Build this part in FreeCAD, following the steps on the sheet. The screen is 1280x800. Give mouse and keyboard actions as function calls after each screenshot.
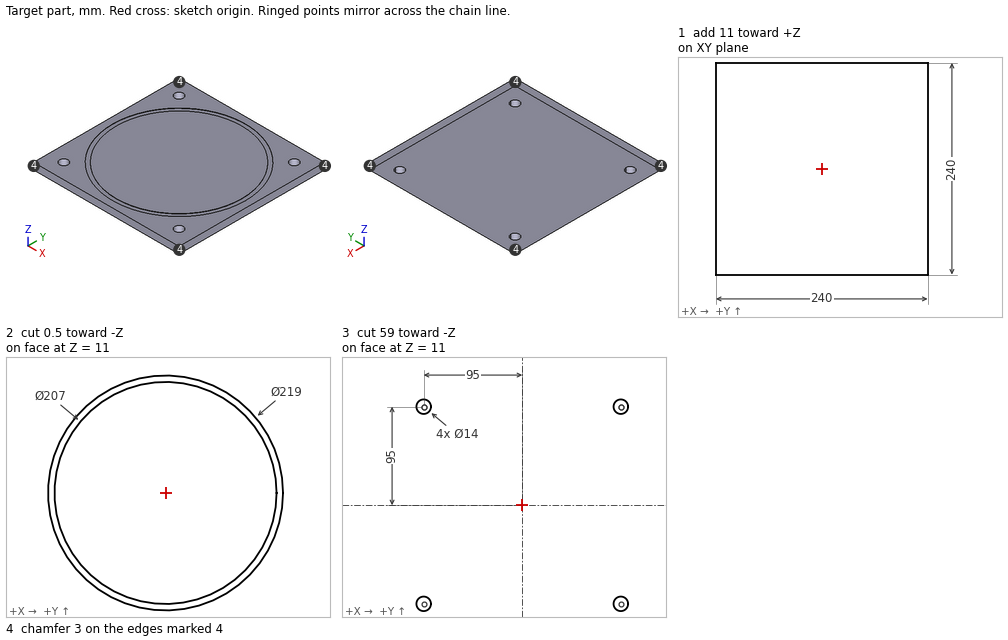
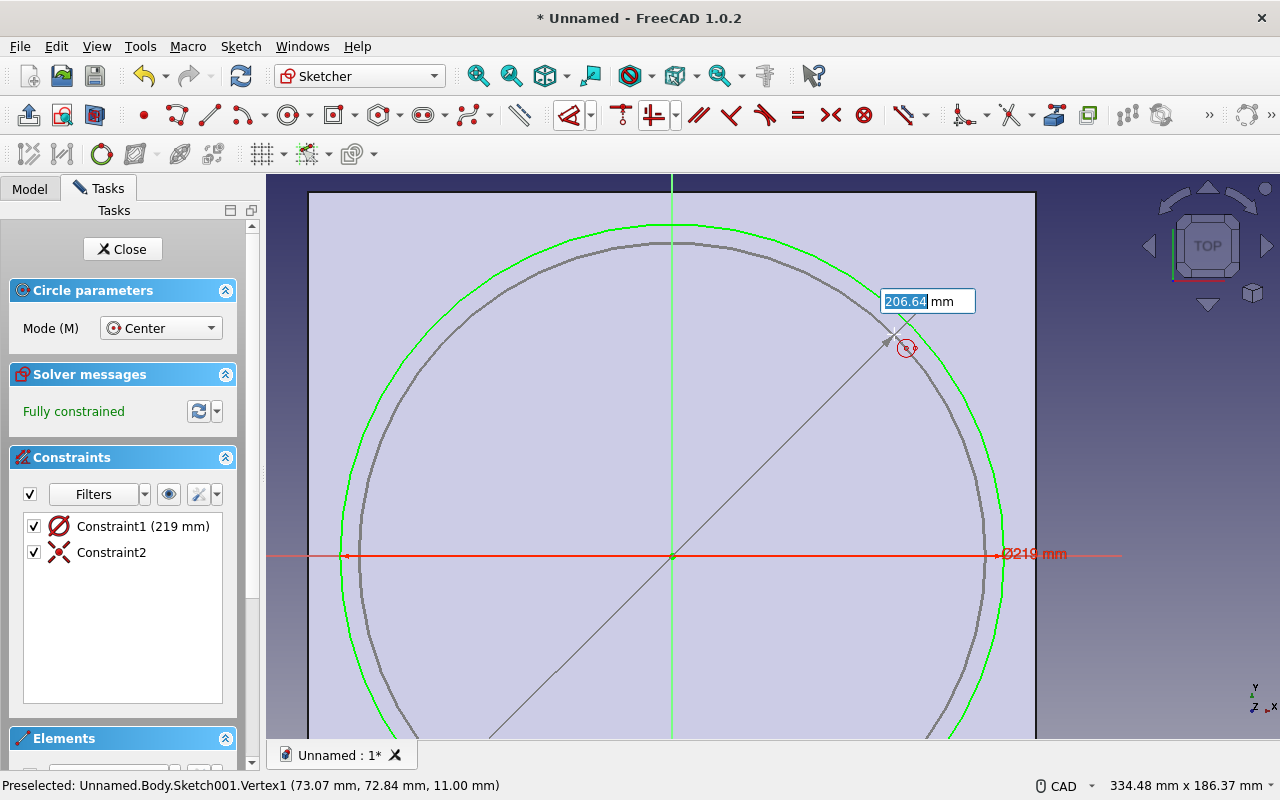
text(207)
key(Return)
key(Escape)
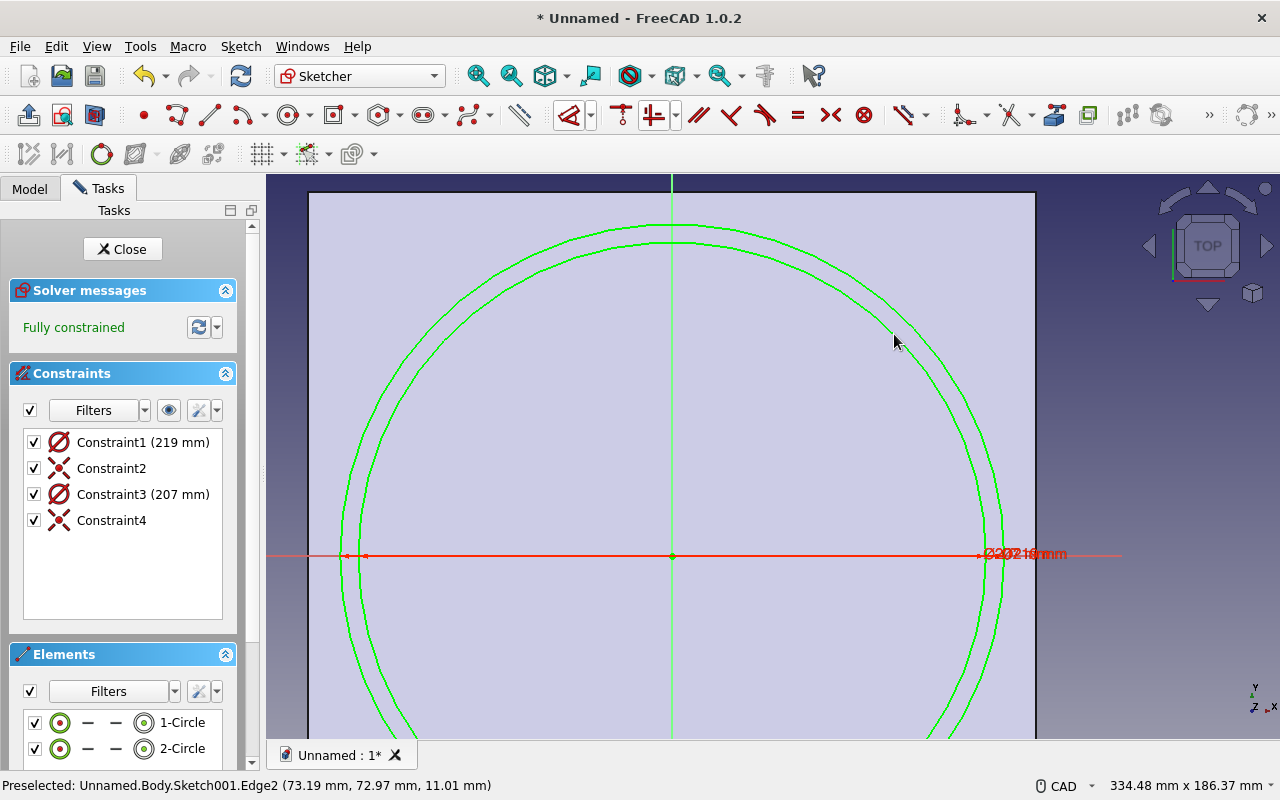
click(123, 249)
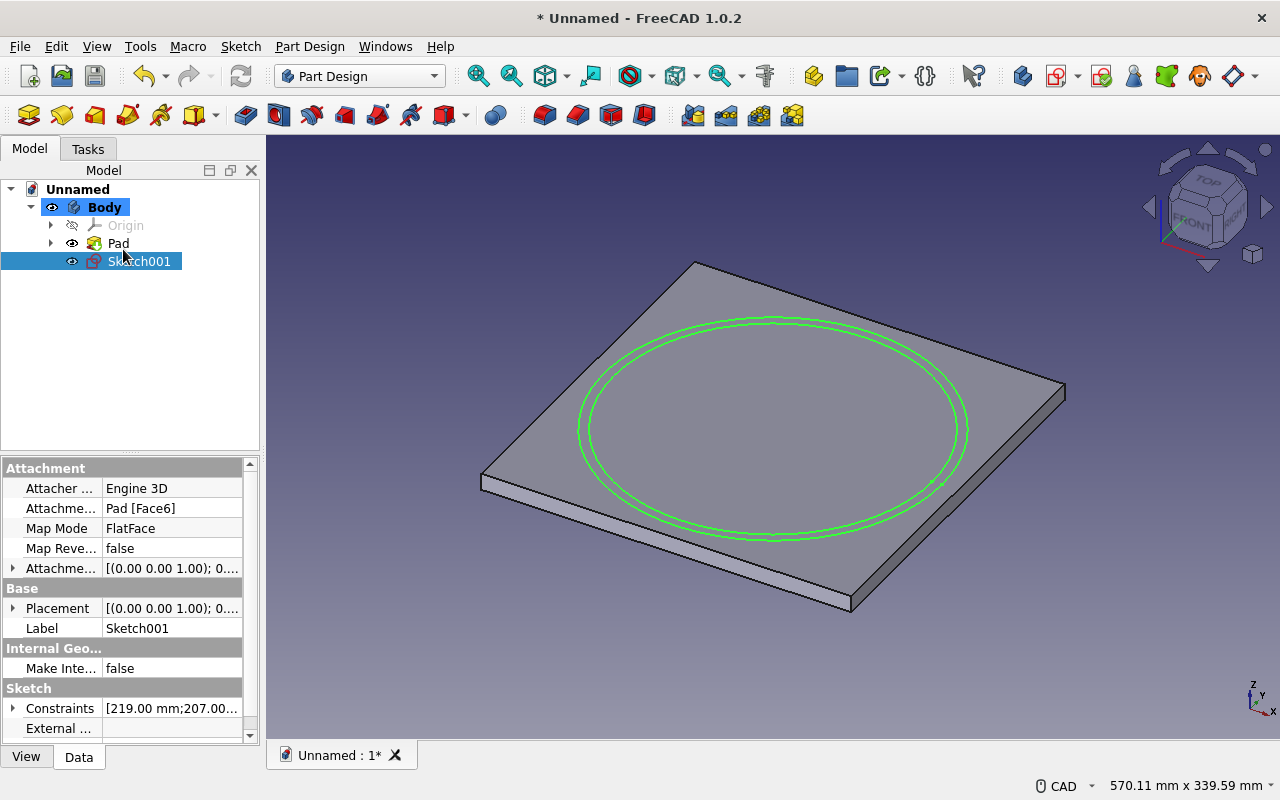
click(246, 116)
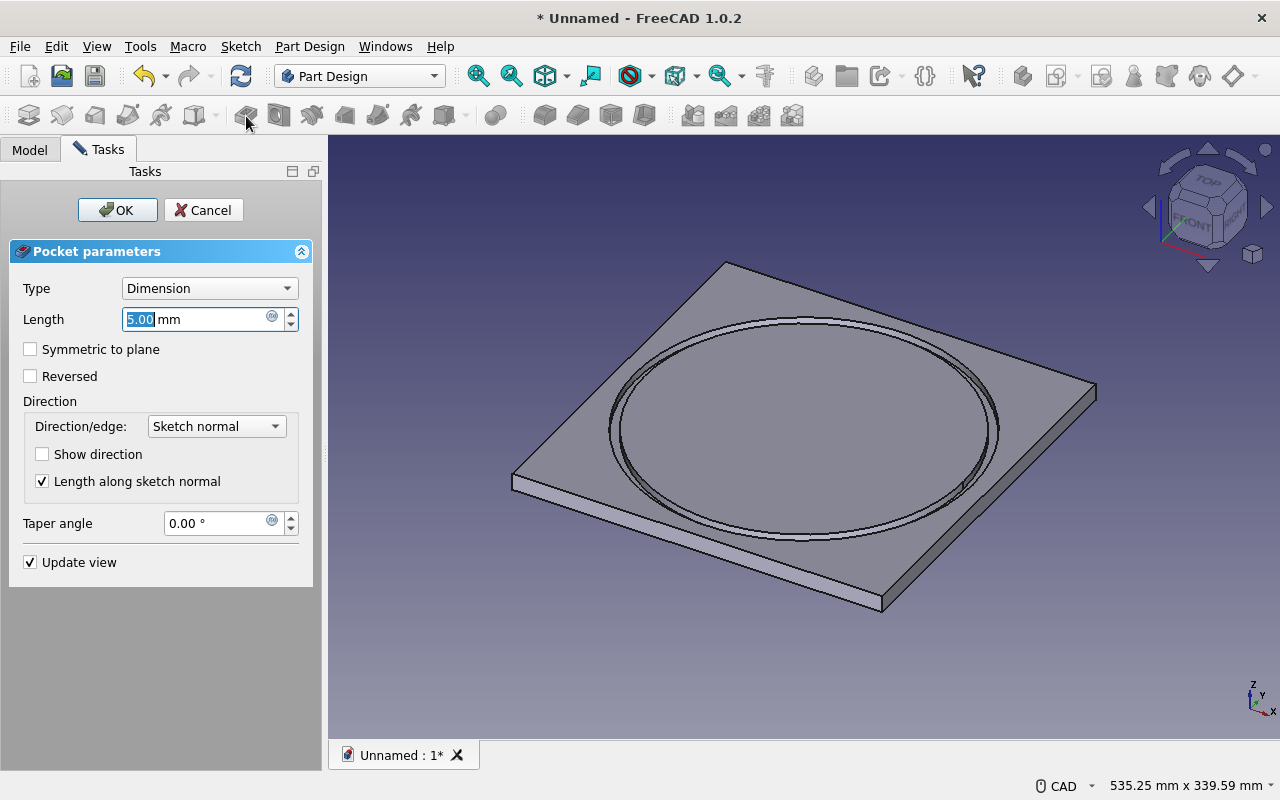
text(0.5)
key(Tab)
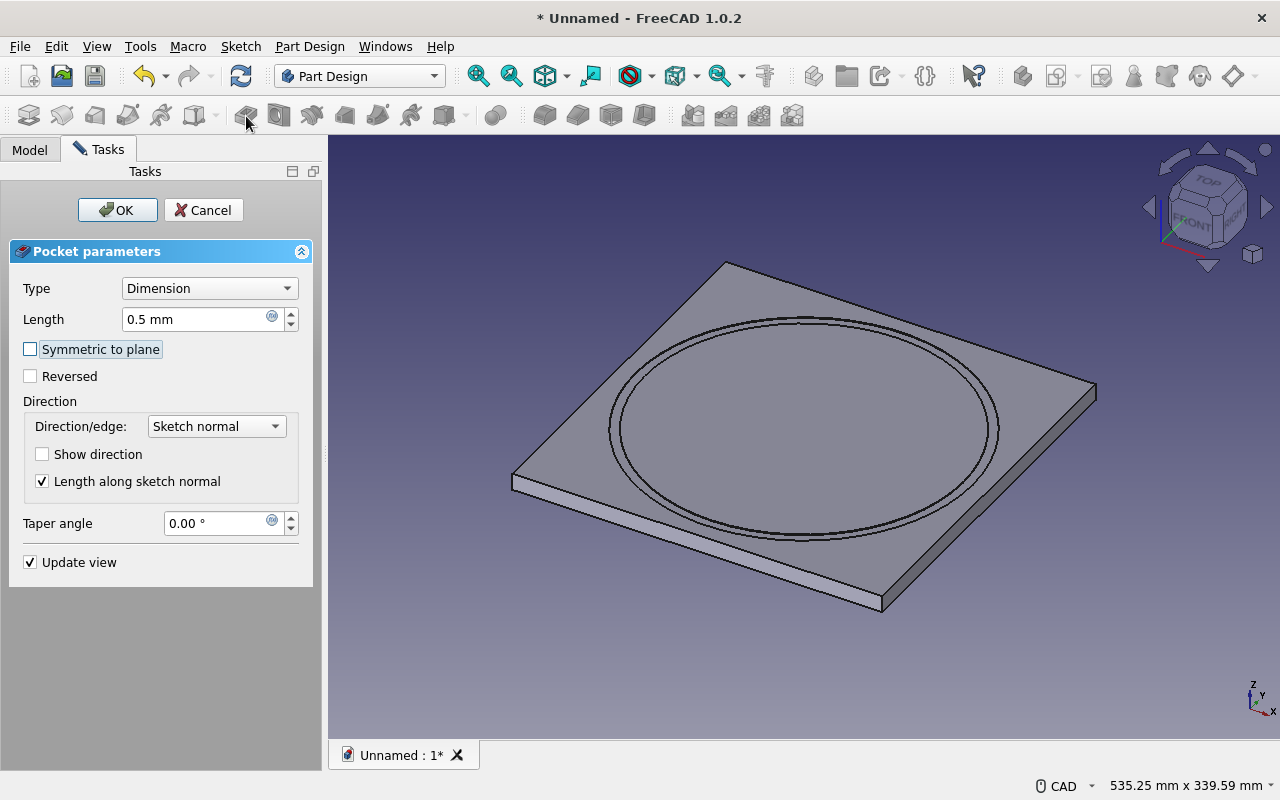
click(118, 210)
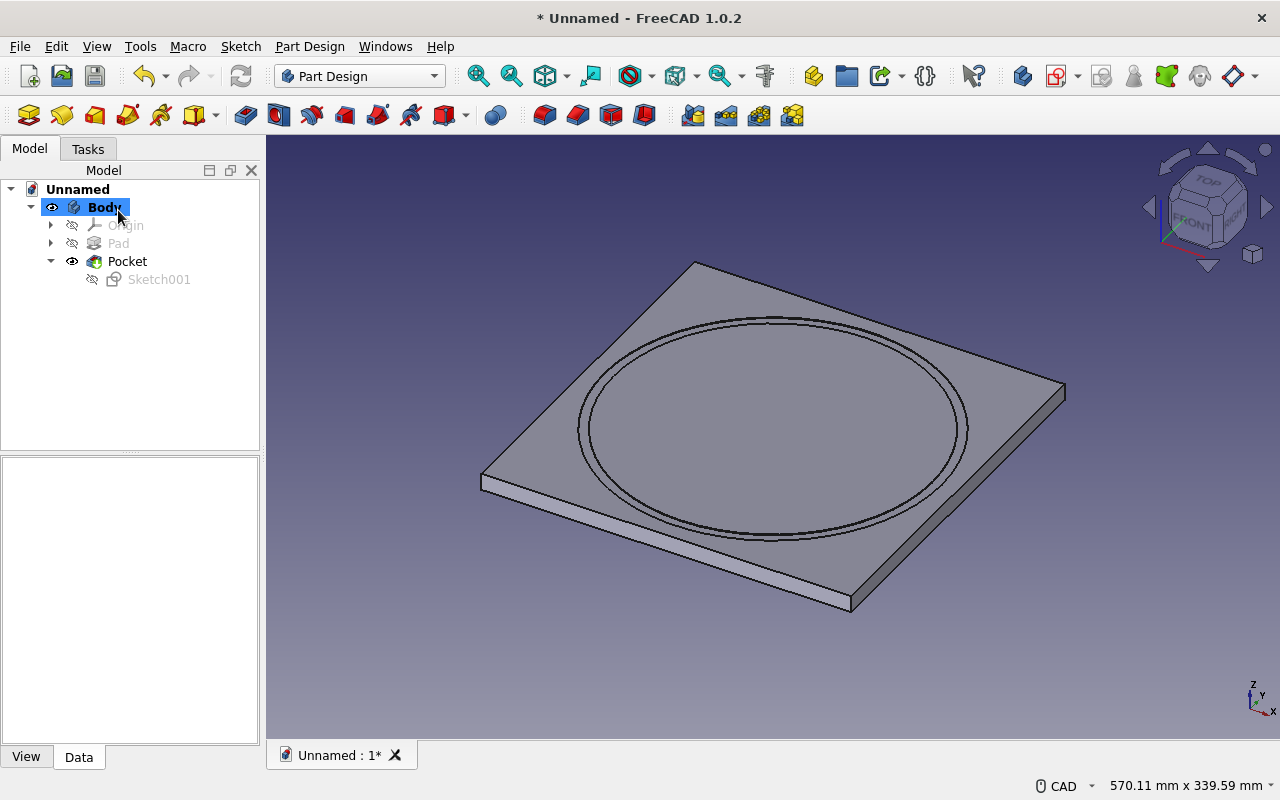
click(773, 428)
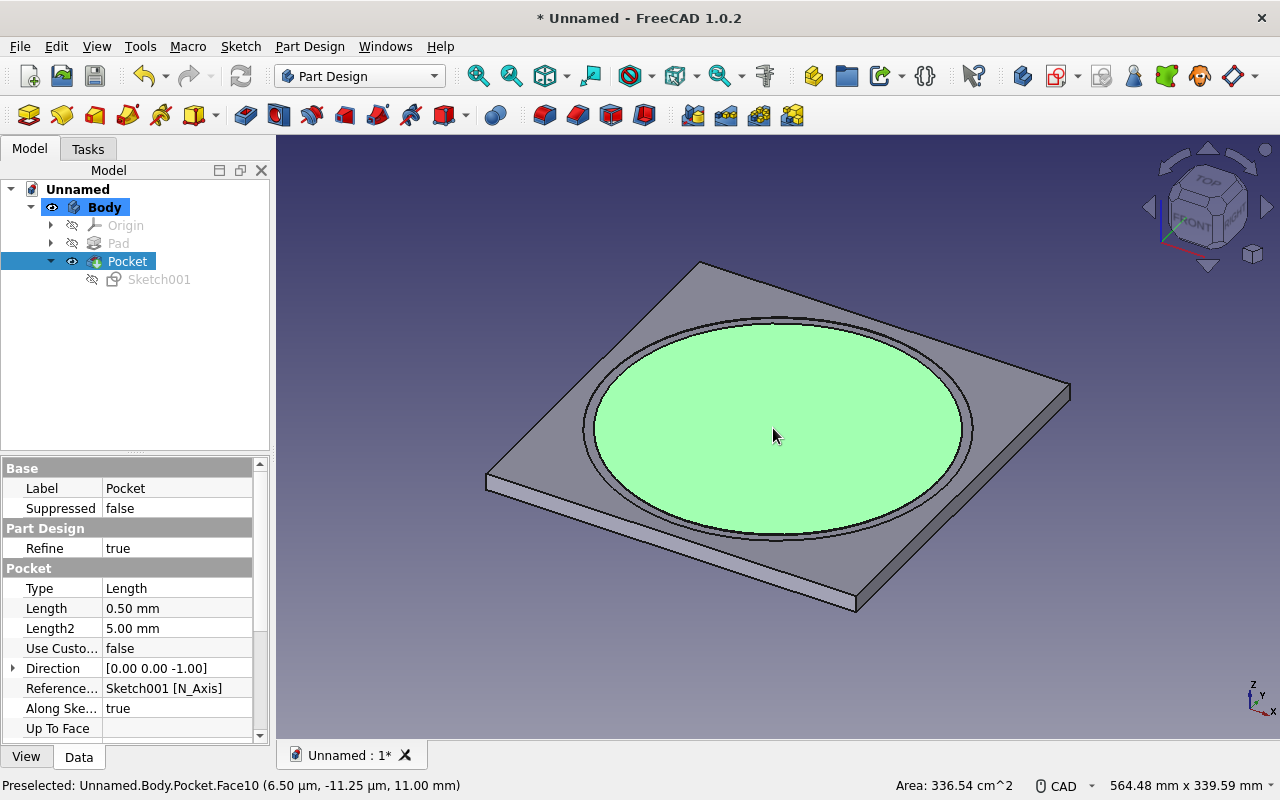
click(1056, 76)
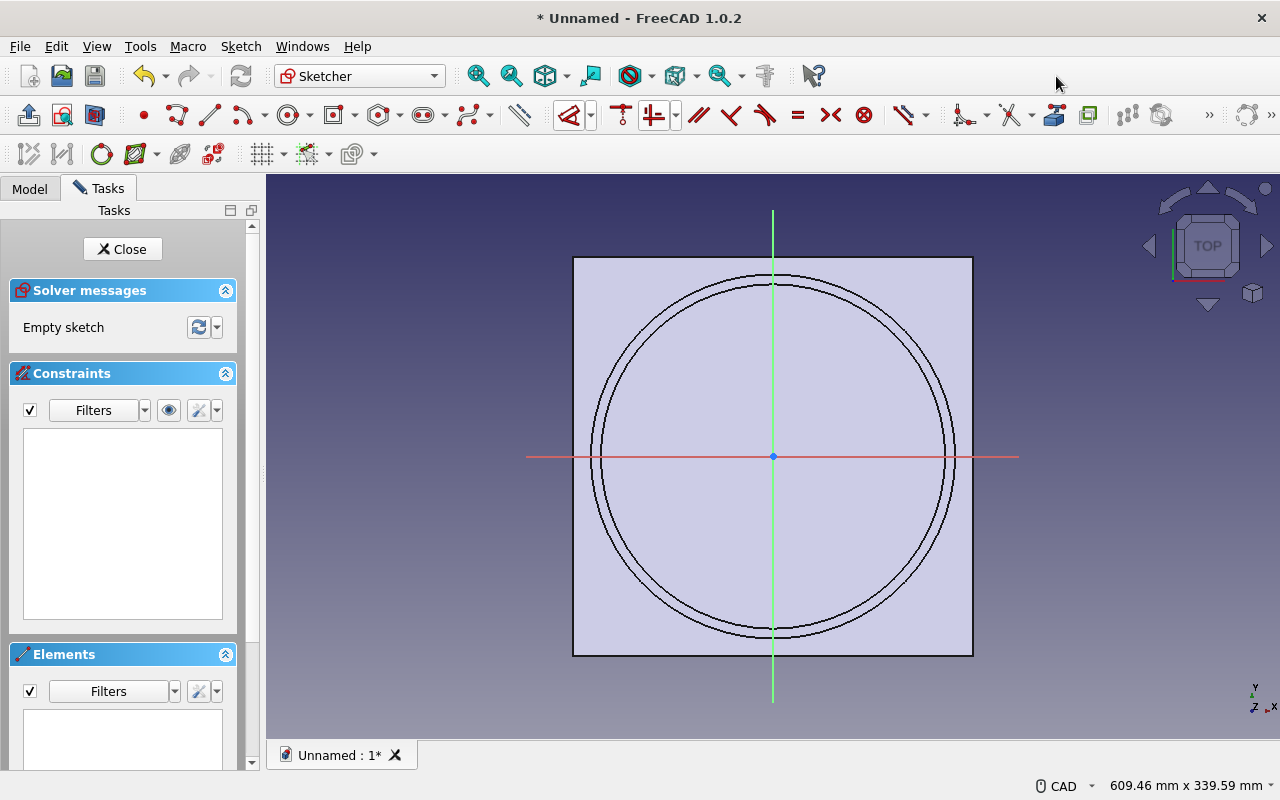
click(288, 116)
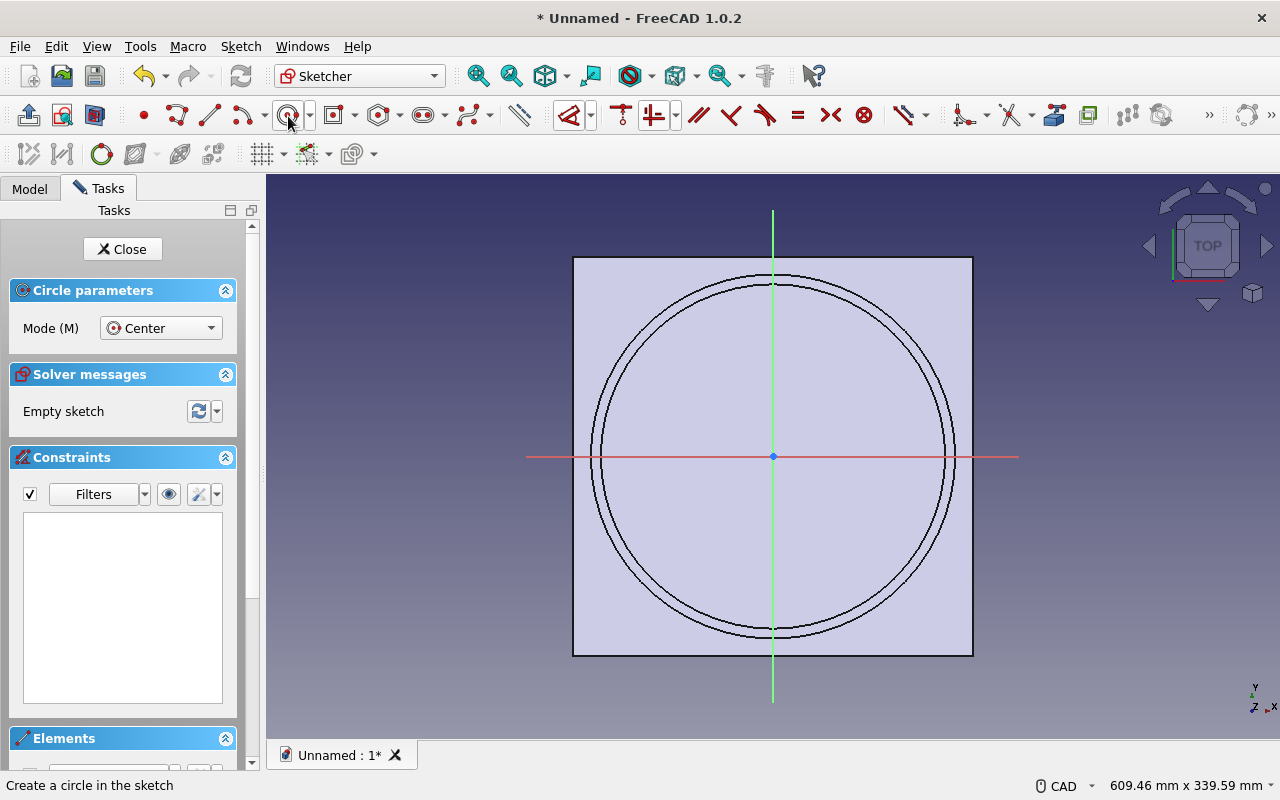
scroll(615, 298, up, 4)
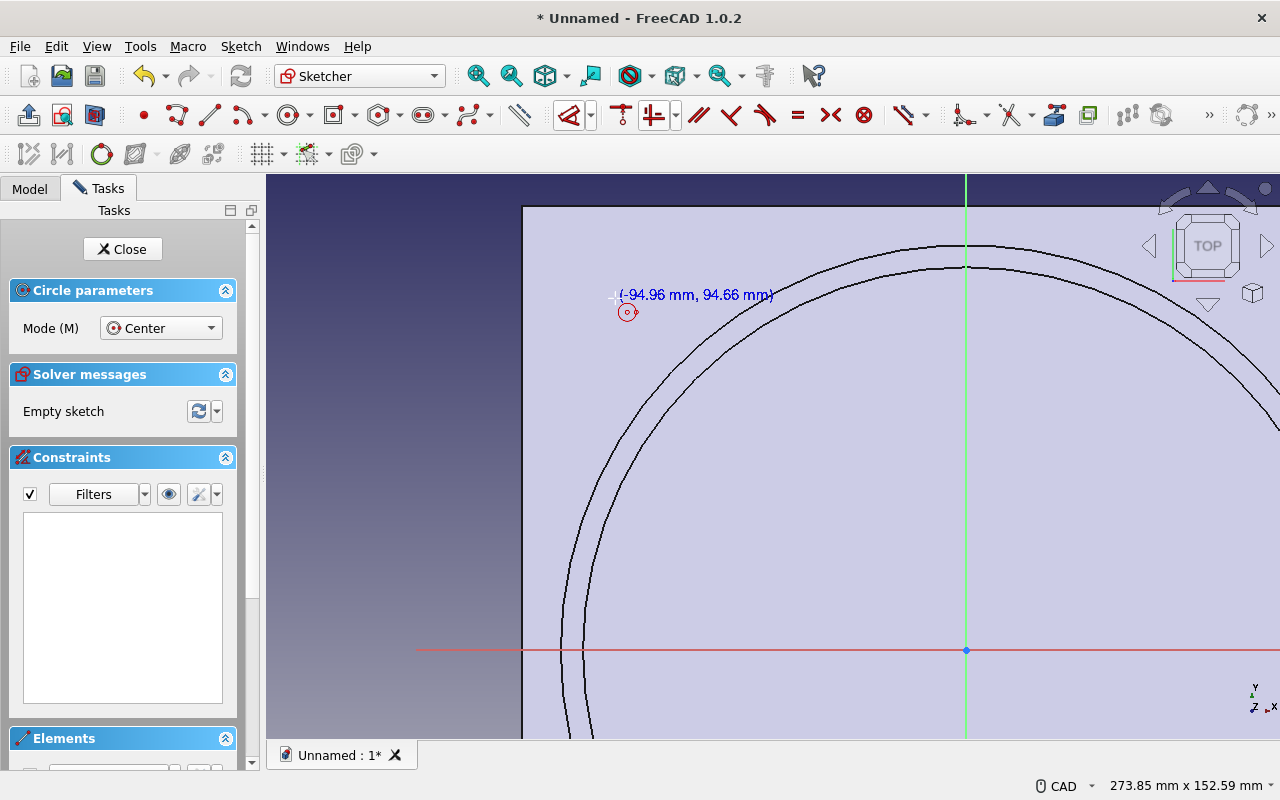
click(614, 299)
move(633, 280)